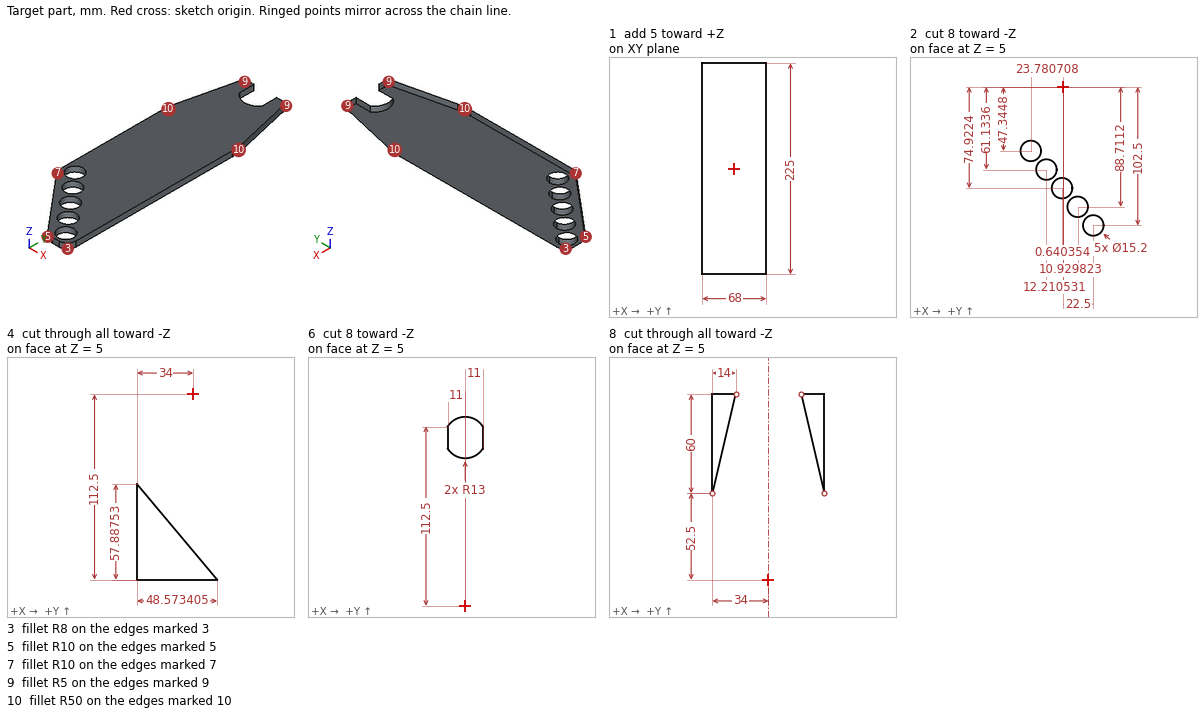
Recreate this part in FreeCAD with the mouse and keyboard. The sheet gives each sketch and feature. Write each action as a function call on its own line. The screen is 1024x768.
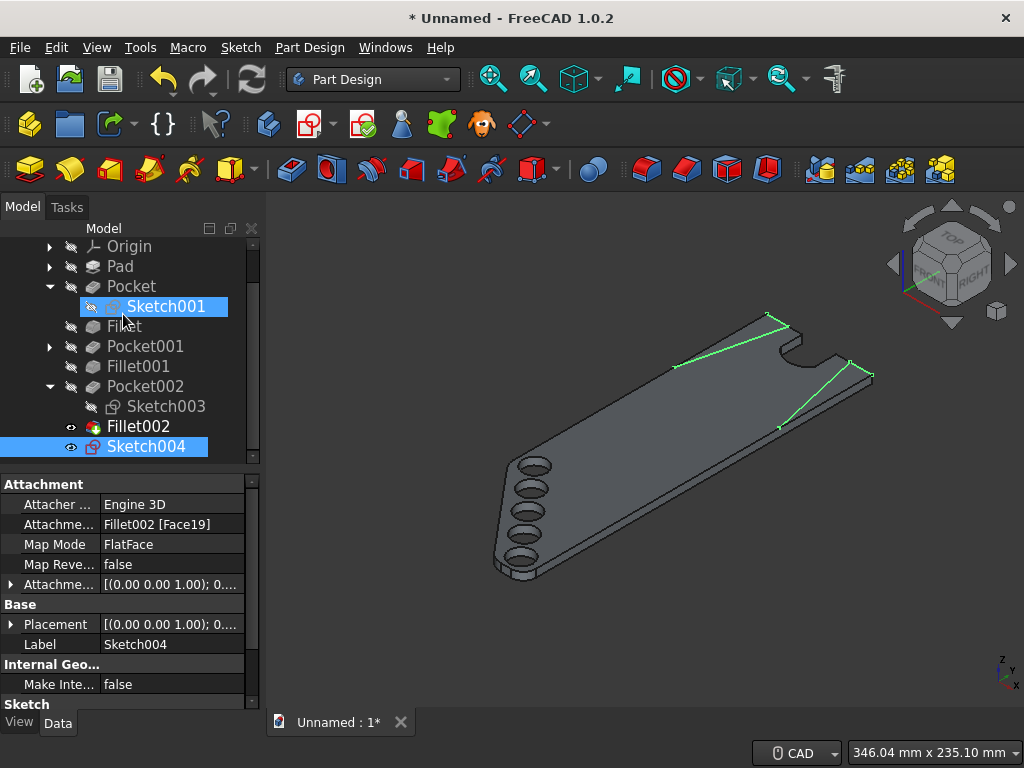
click(292, 170)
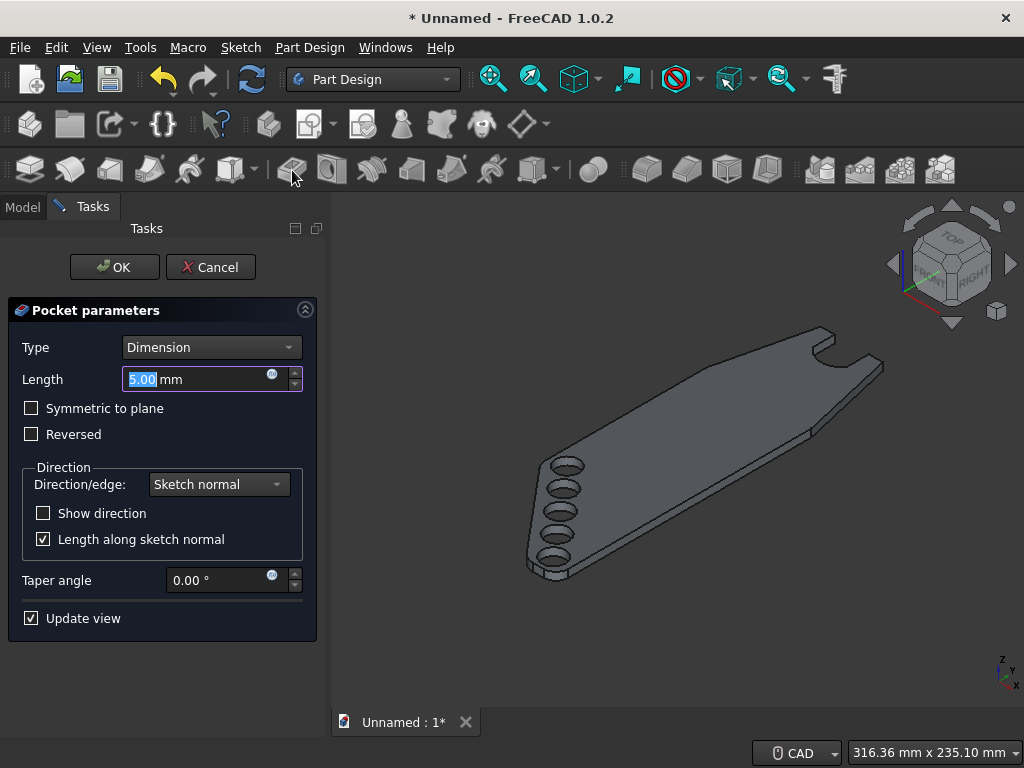
click(212, 348)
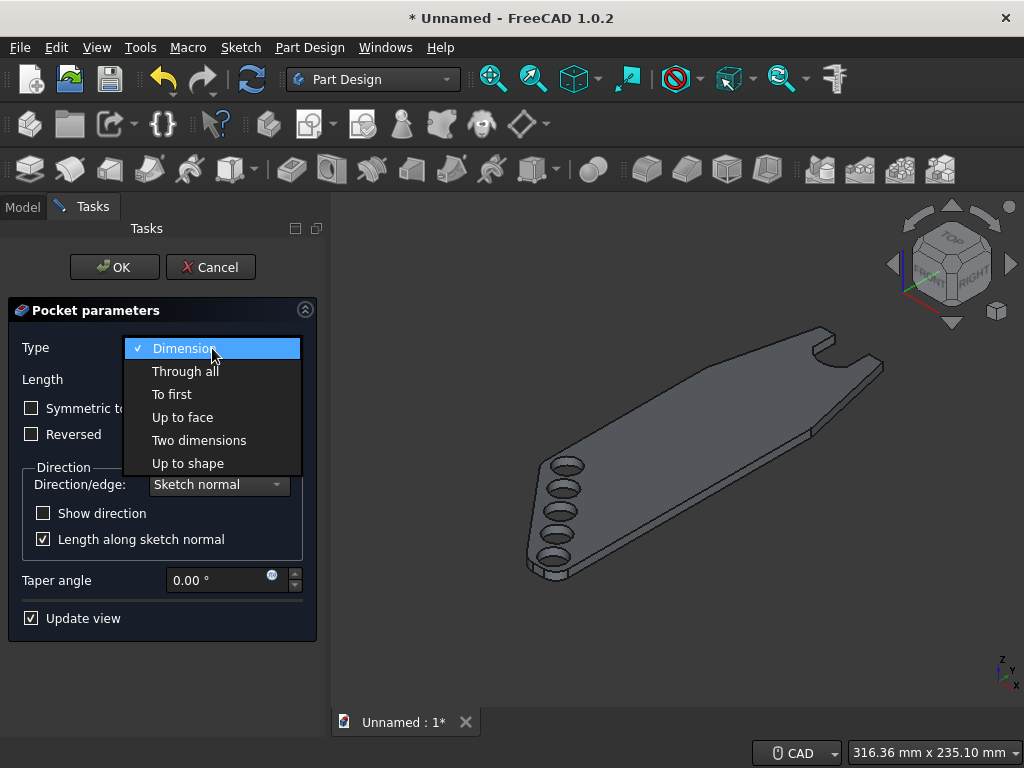
click(212, 372)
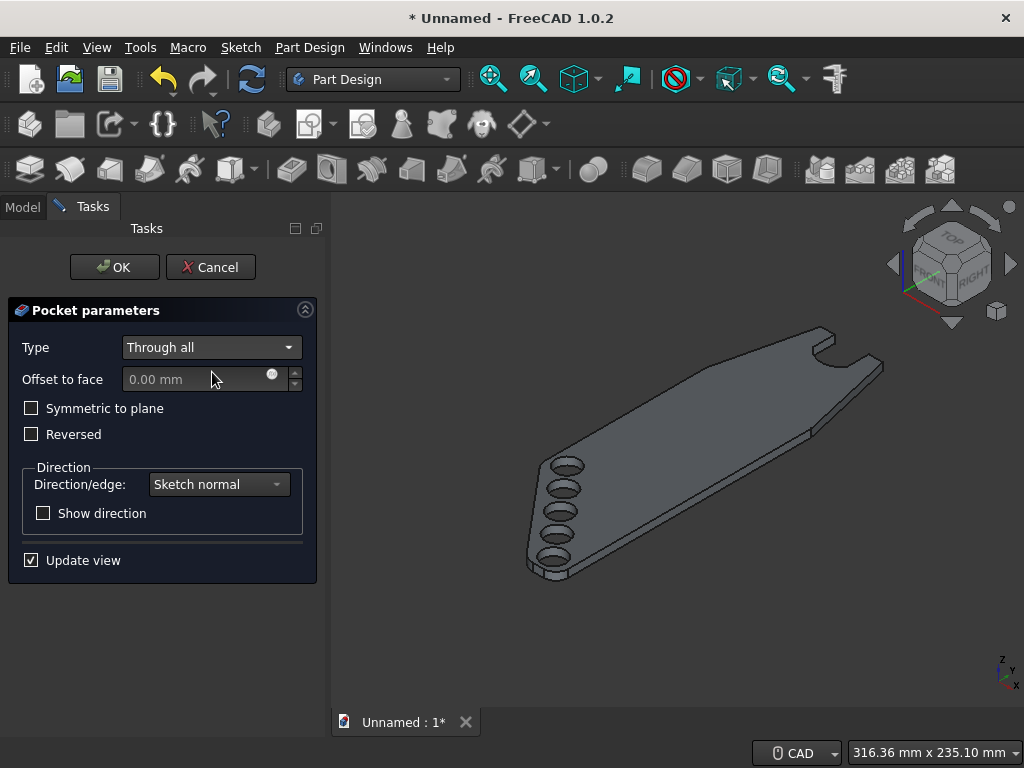
click(115, 267)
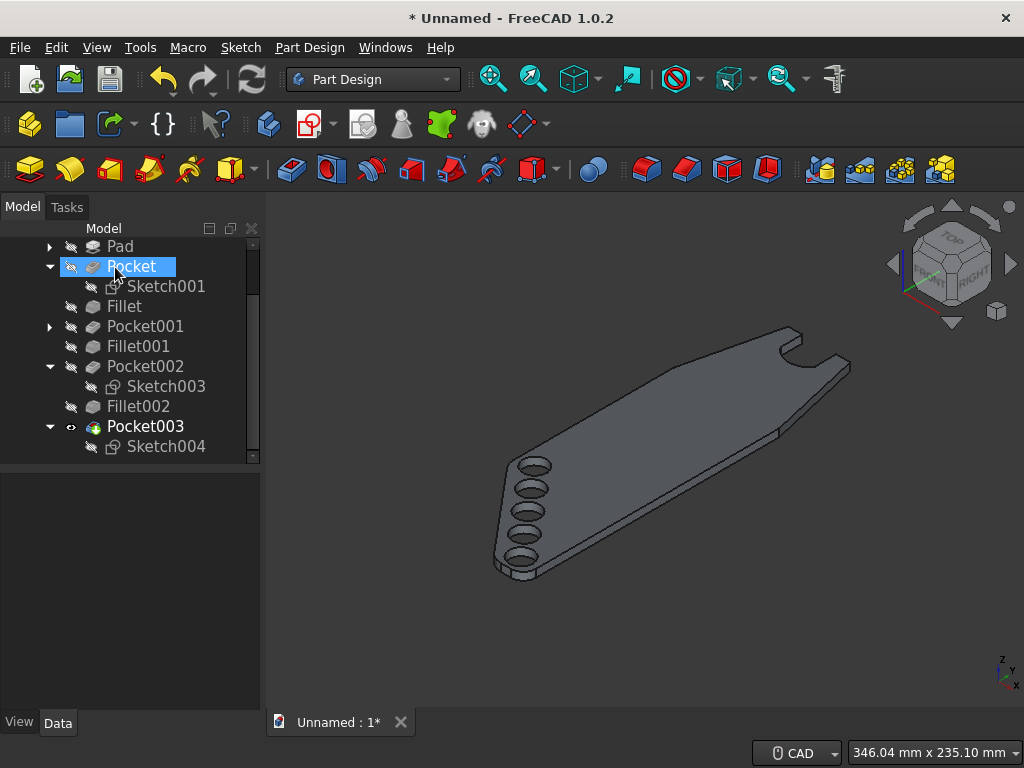
scroll(850, 366, up, 7)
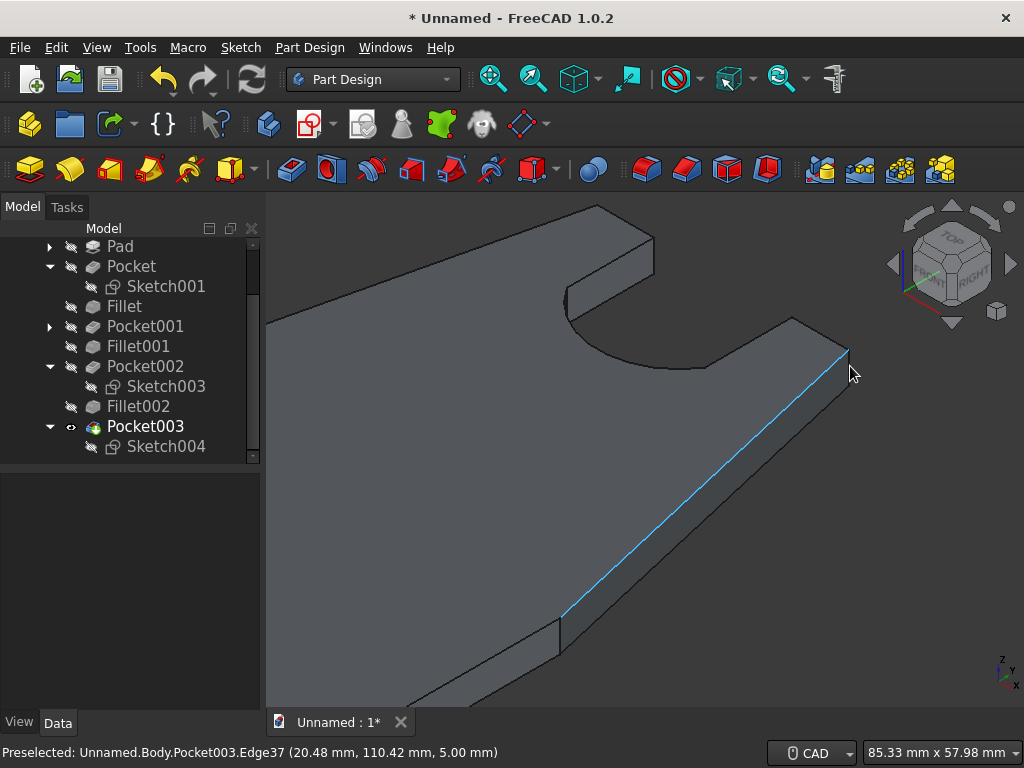
click(494, 80)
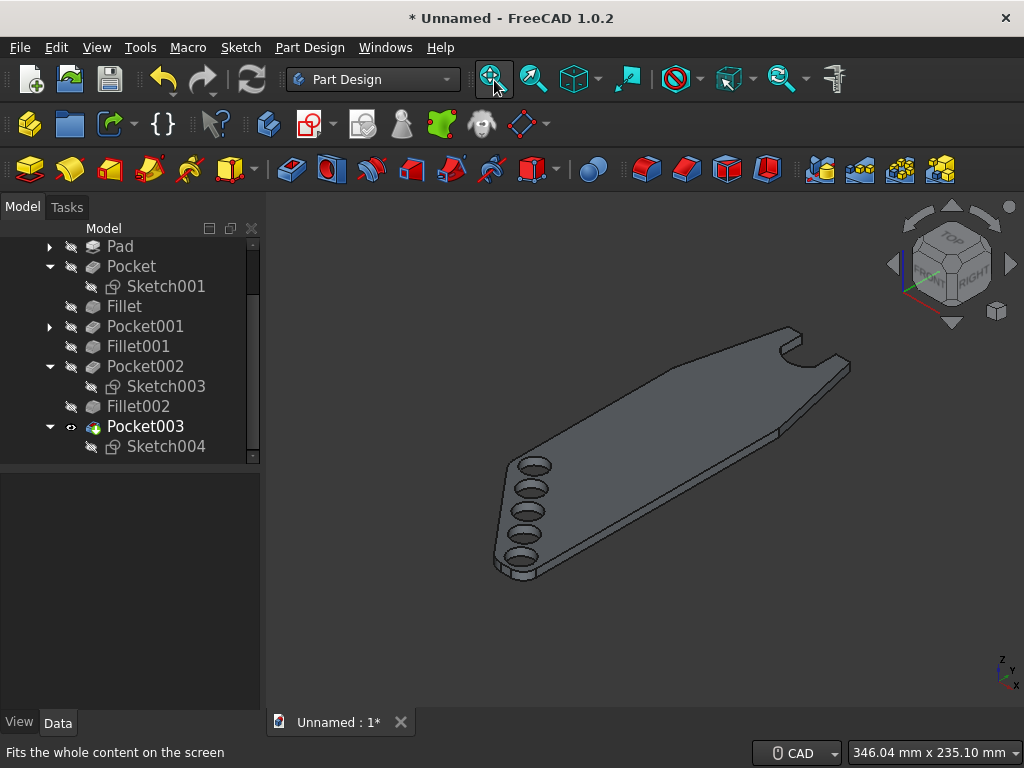
key(2)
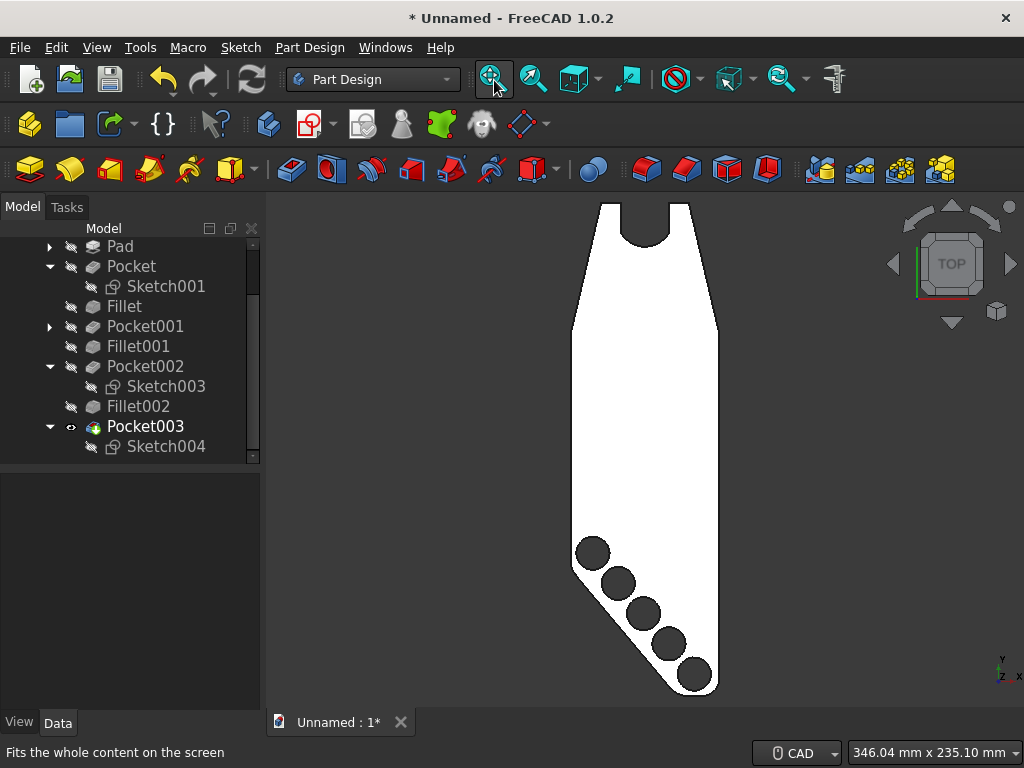
key(0)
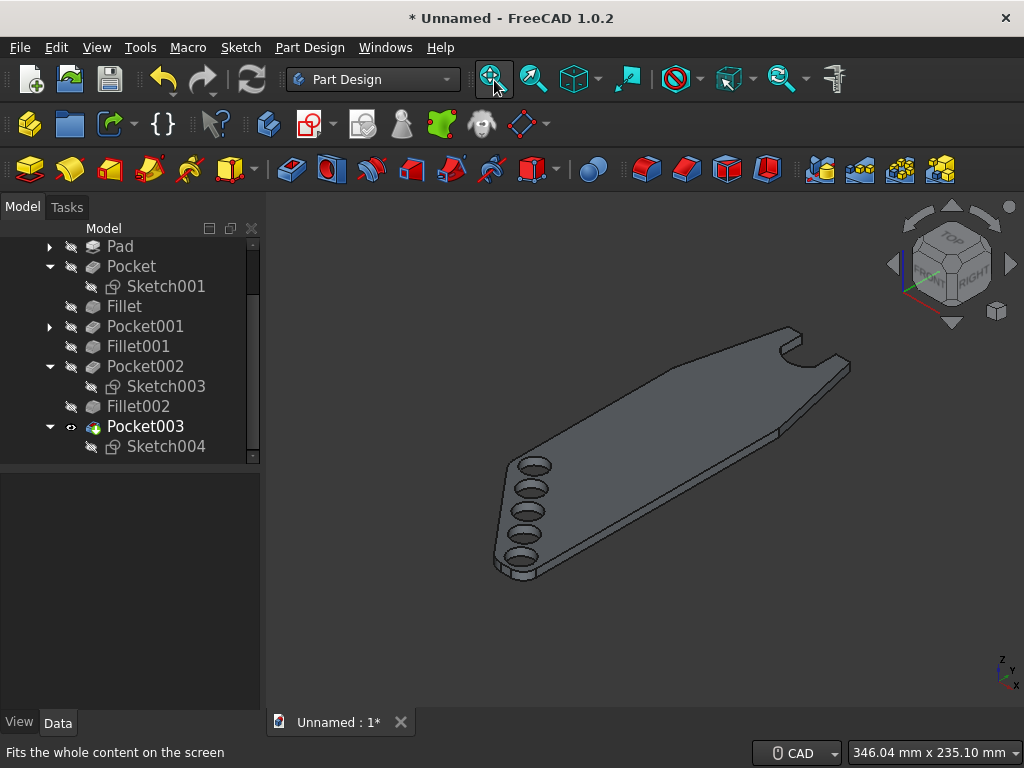
scroll(850, 366, up, 7)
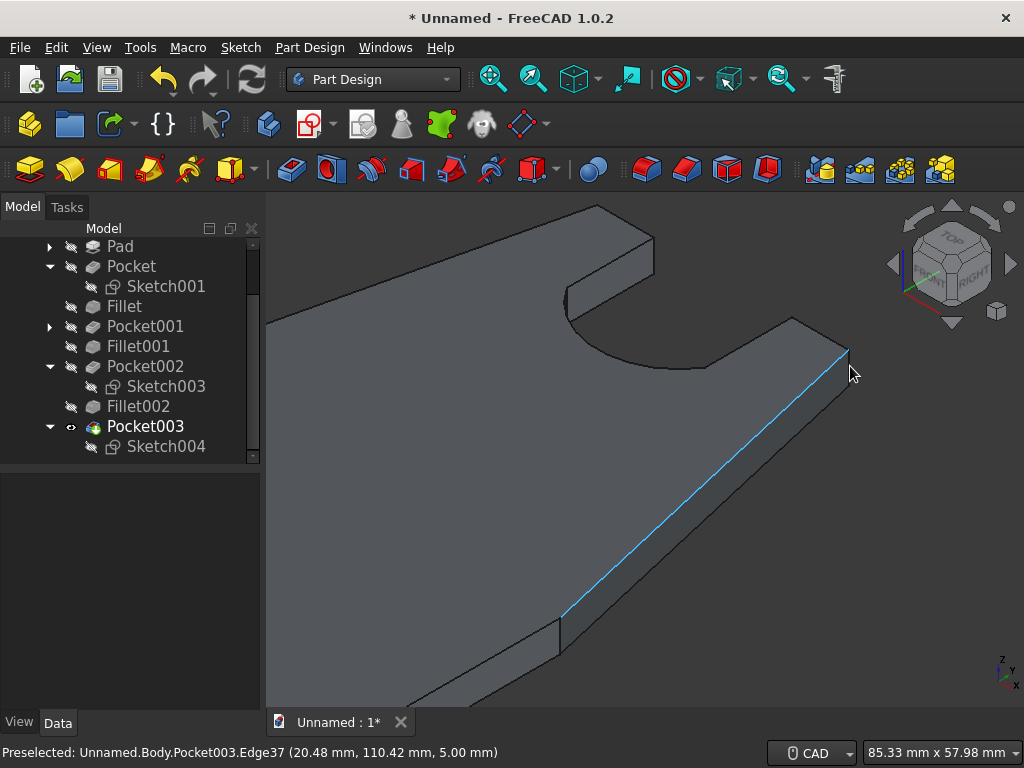
key(v)
key(f)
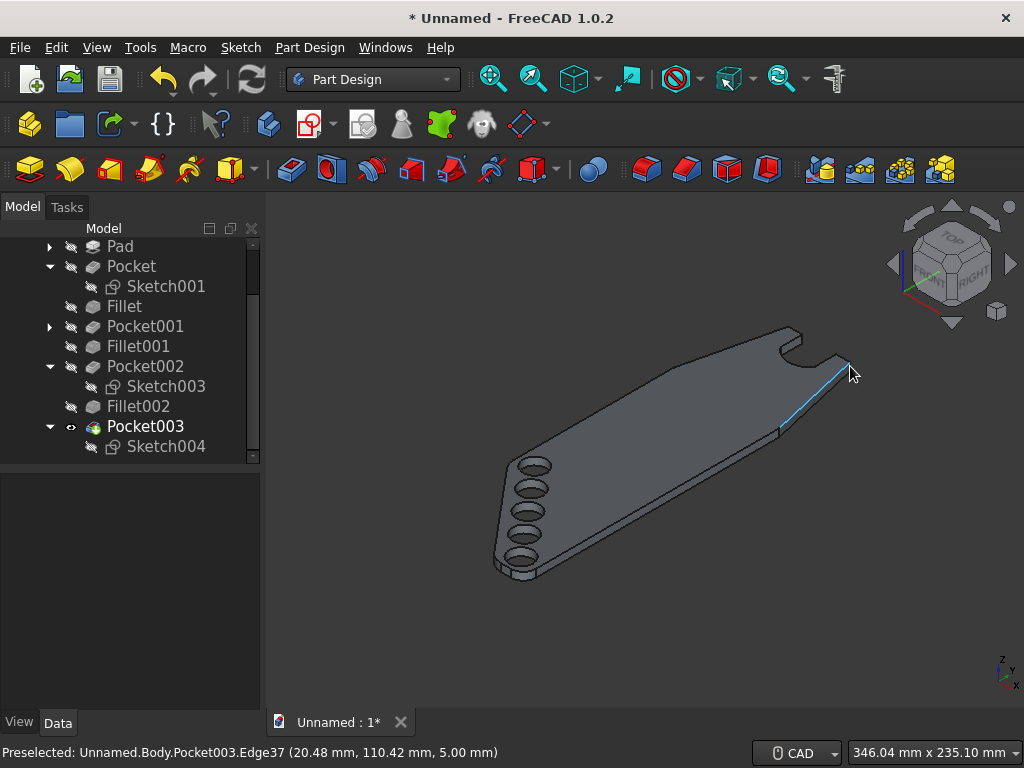
key(1)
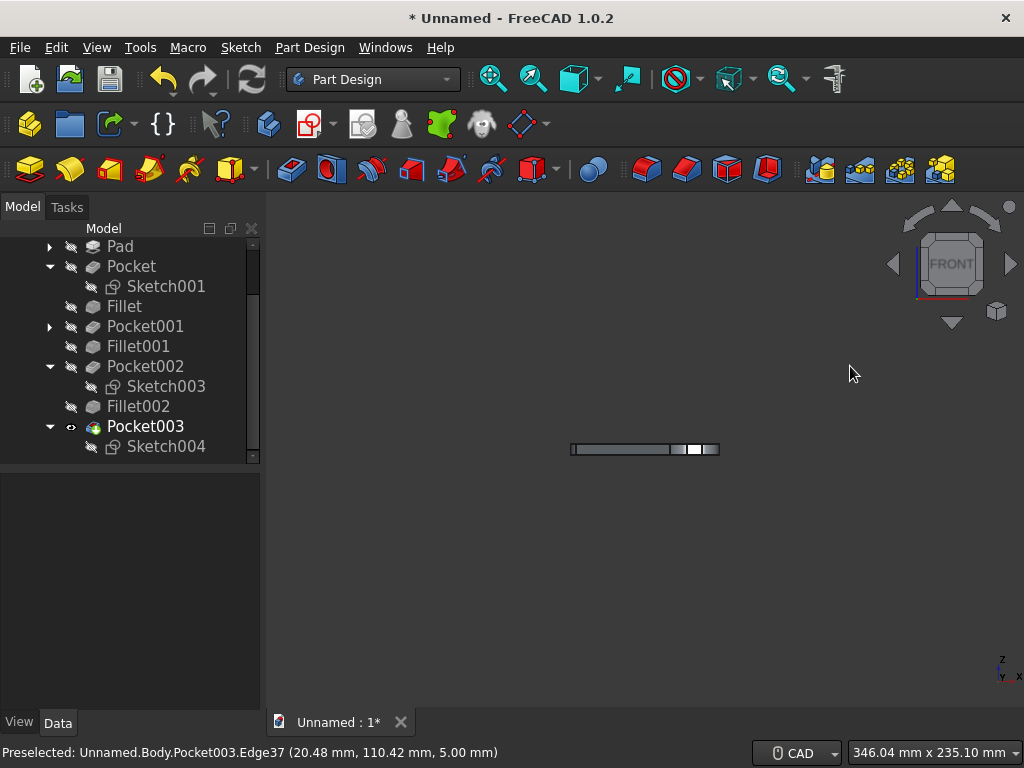
key(v)
key(f)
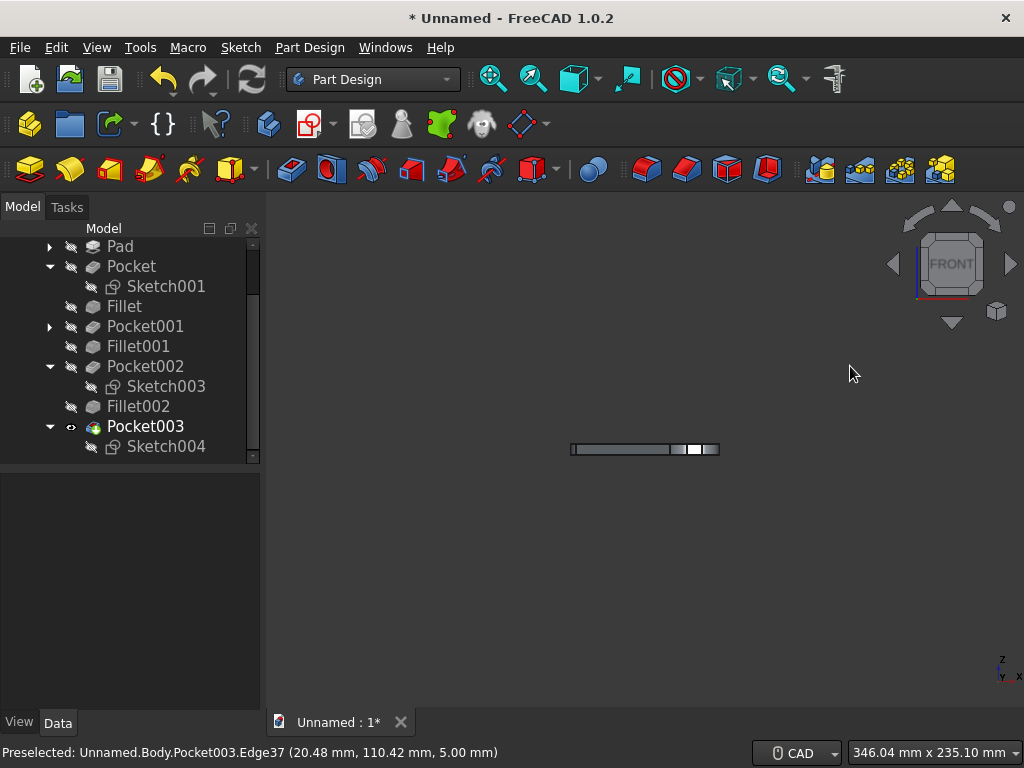
scroll(689, 449, up, 7)